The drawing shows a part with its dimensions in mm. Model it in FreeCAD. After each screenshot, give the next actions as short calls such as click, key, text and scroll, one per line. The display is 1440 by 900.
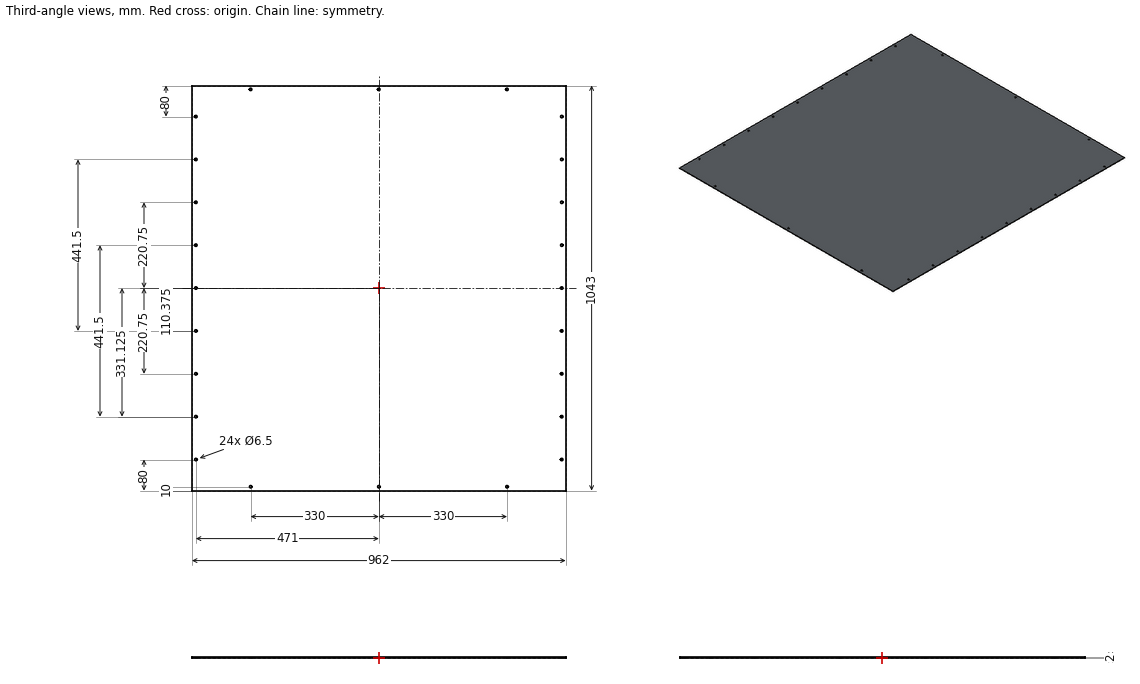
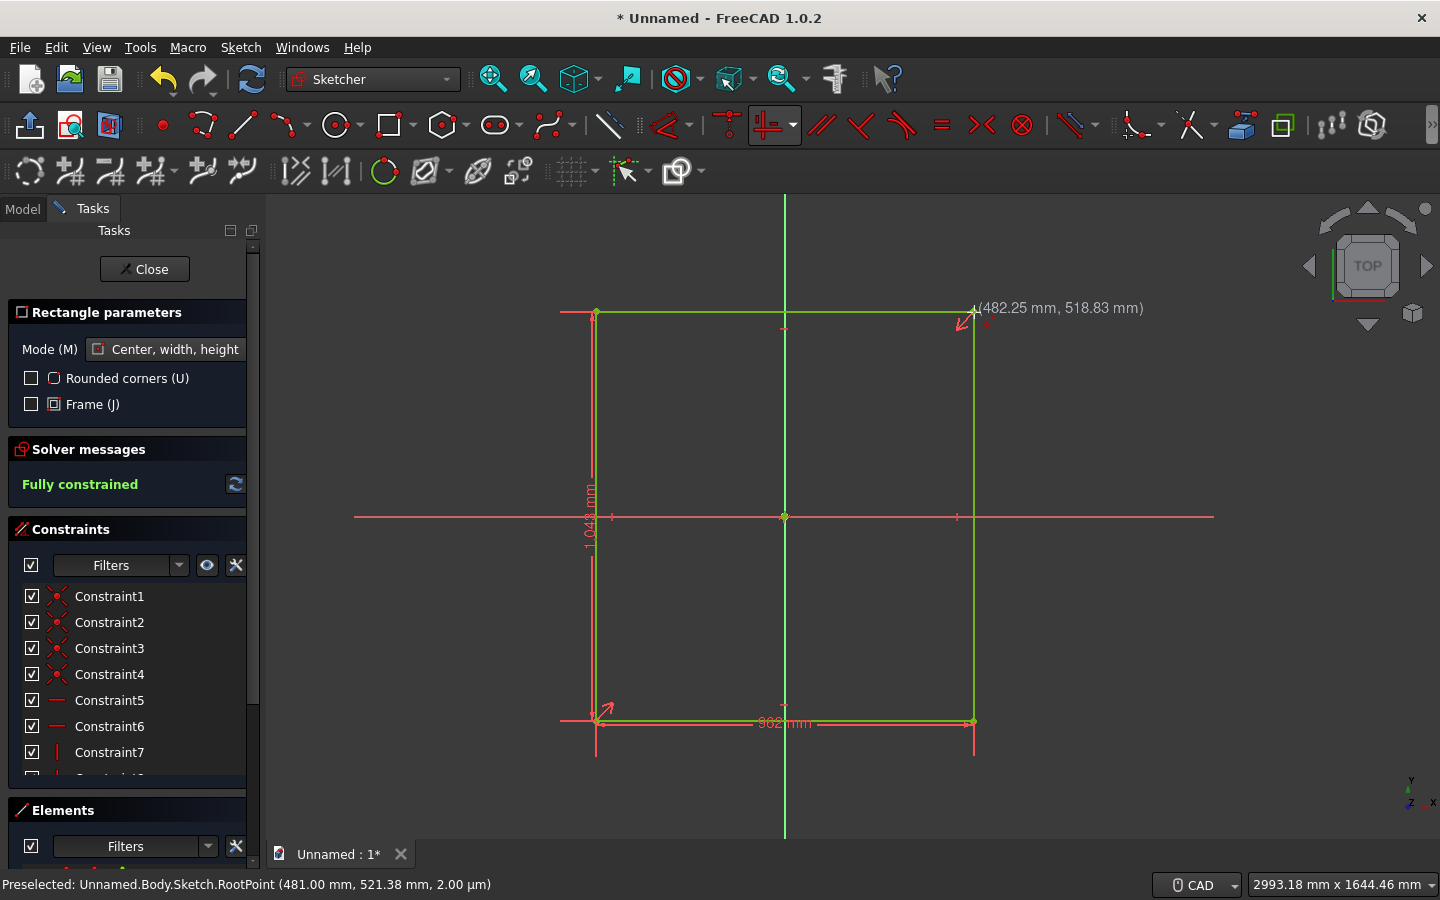
click(336, 126)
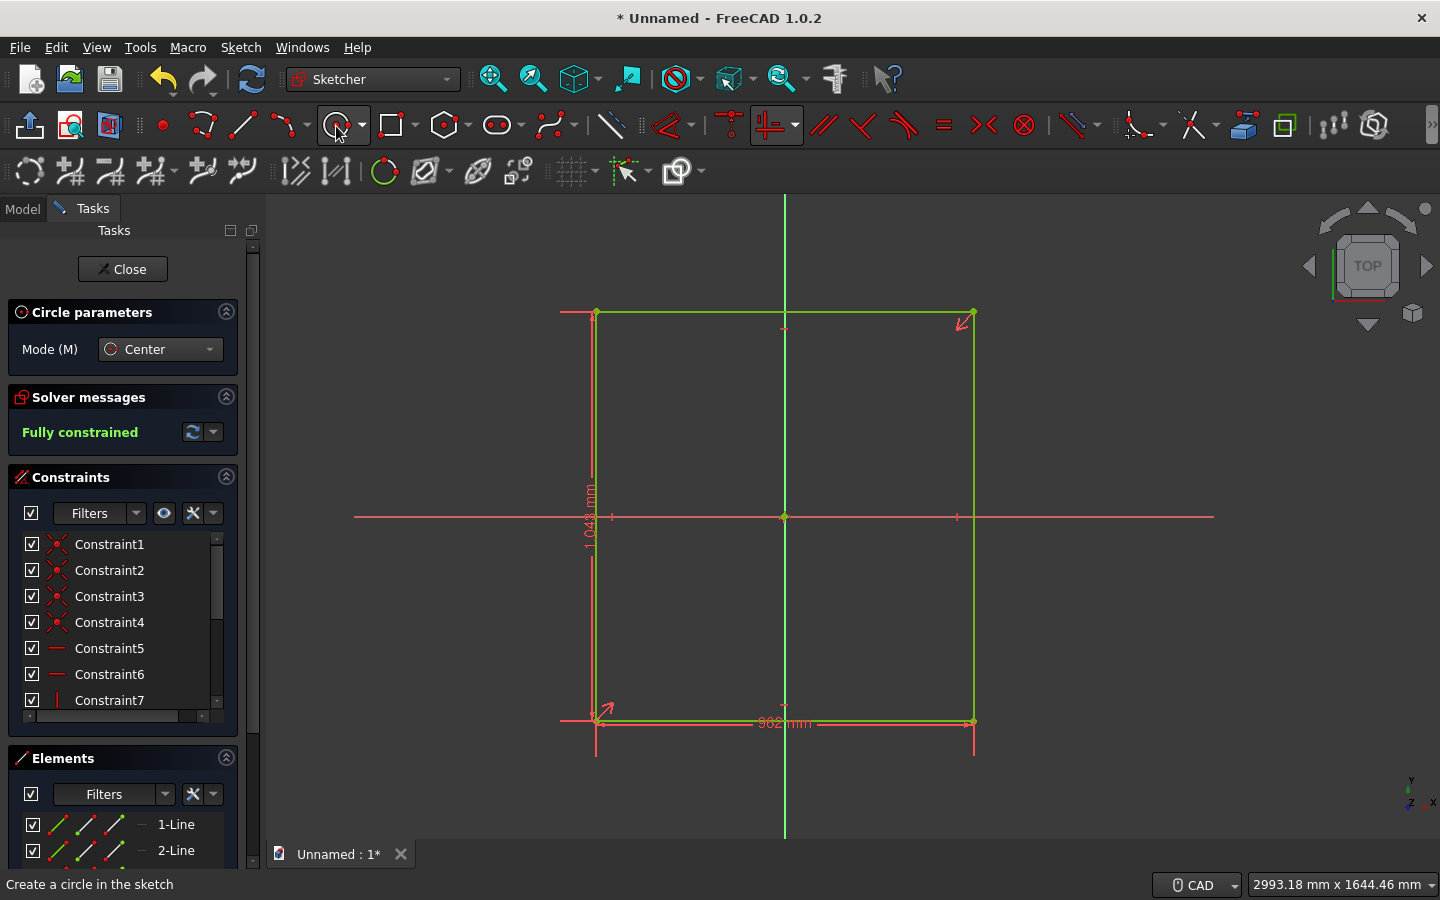
scroll(600, 690, up, 15)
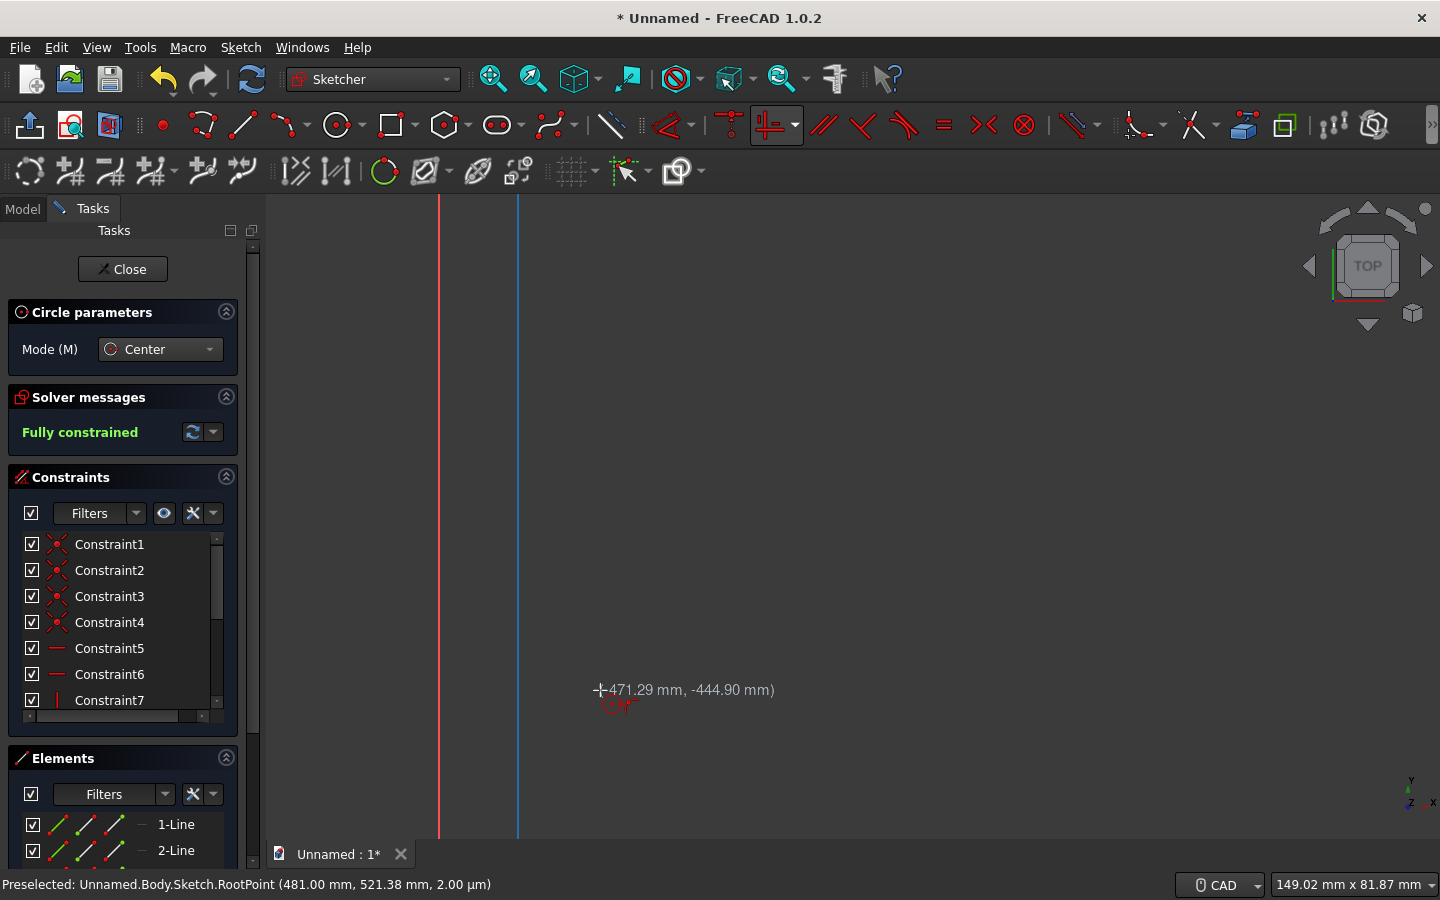
scroll(600, 691, down, 15)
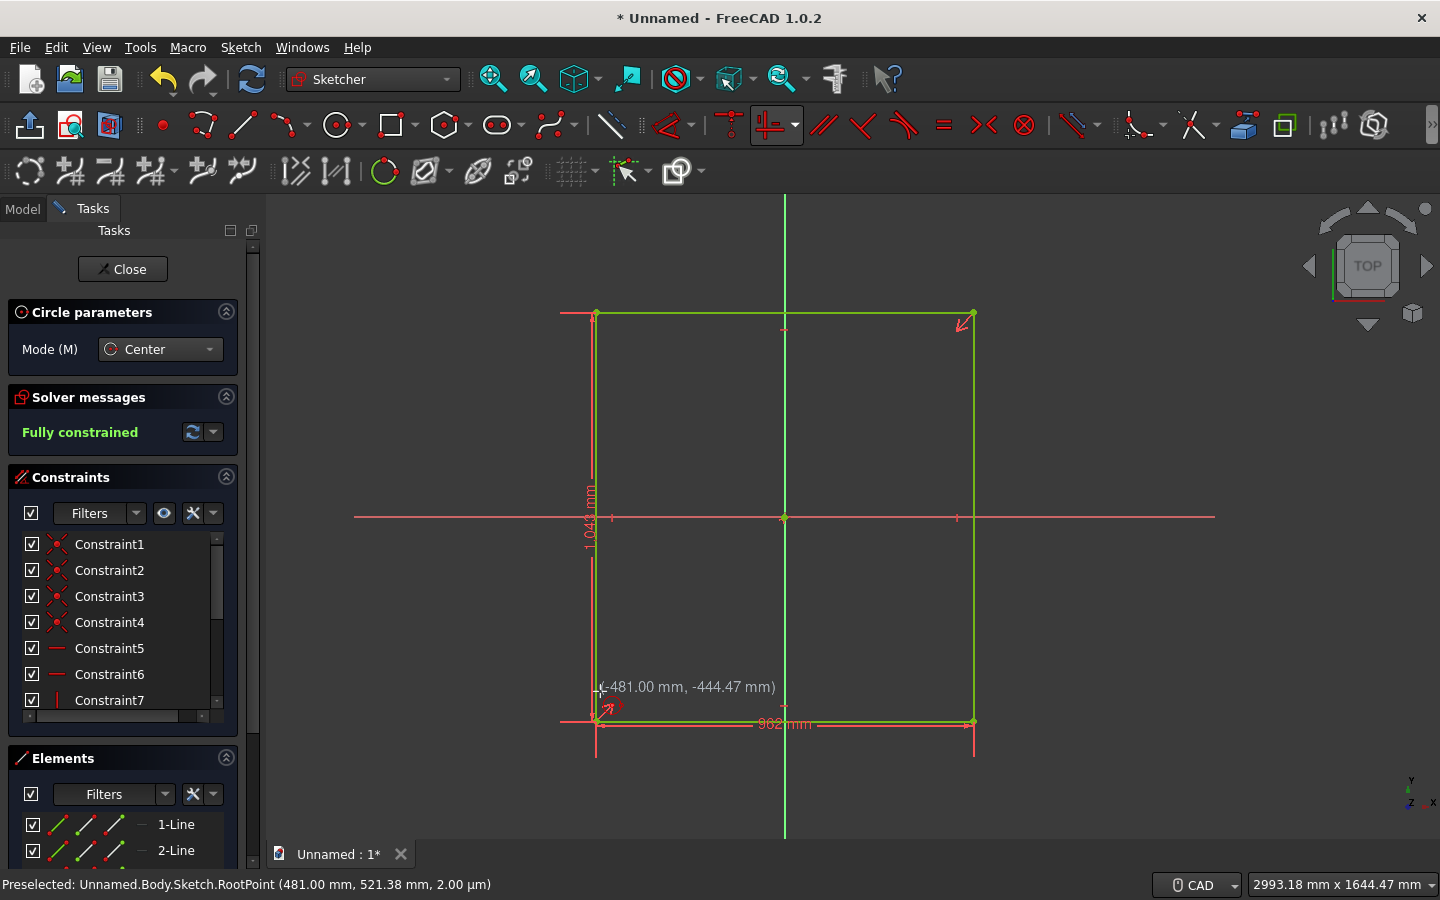
scroll(600, 691, up, 7)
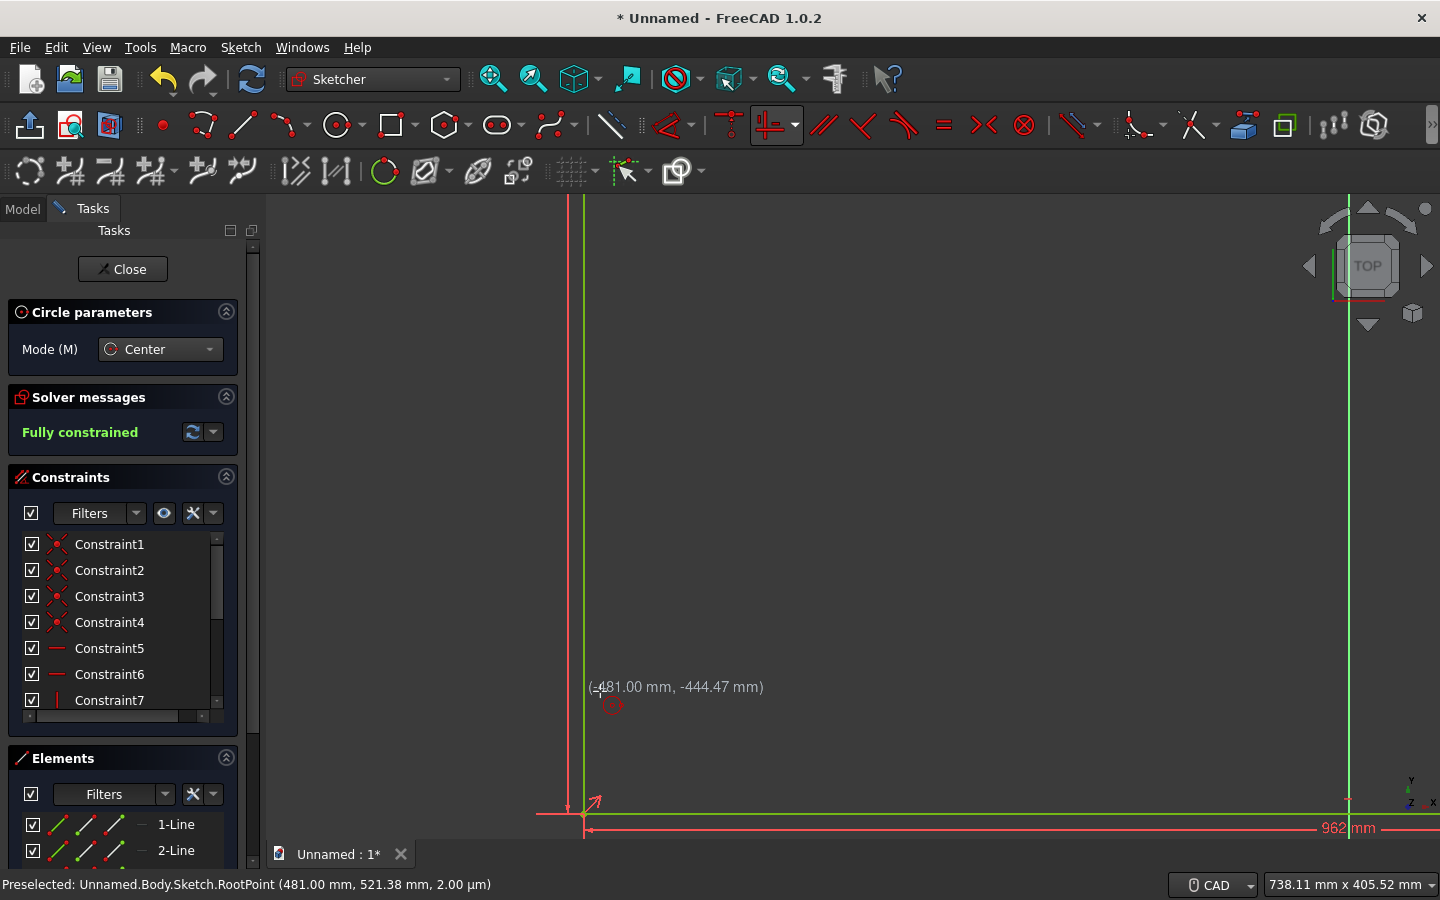
click(600, 687)
move(603, 683)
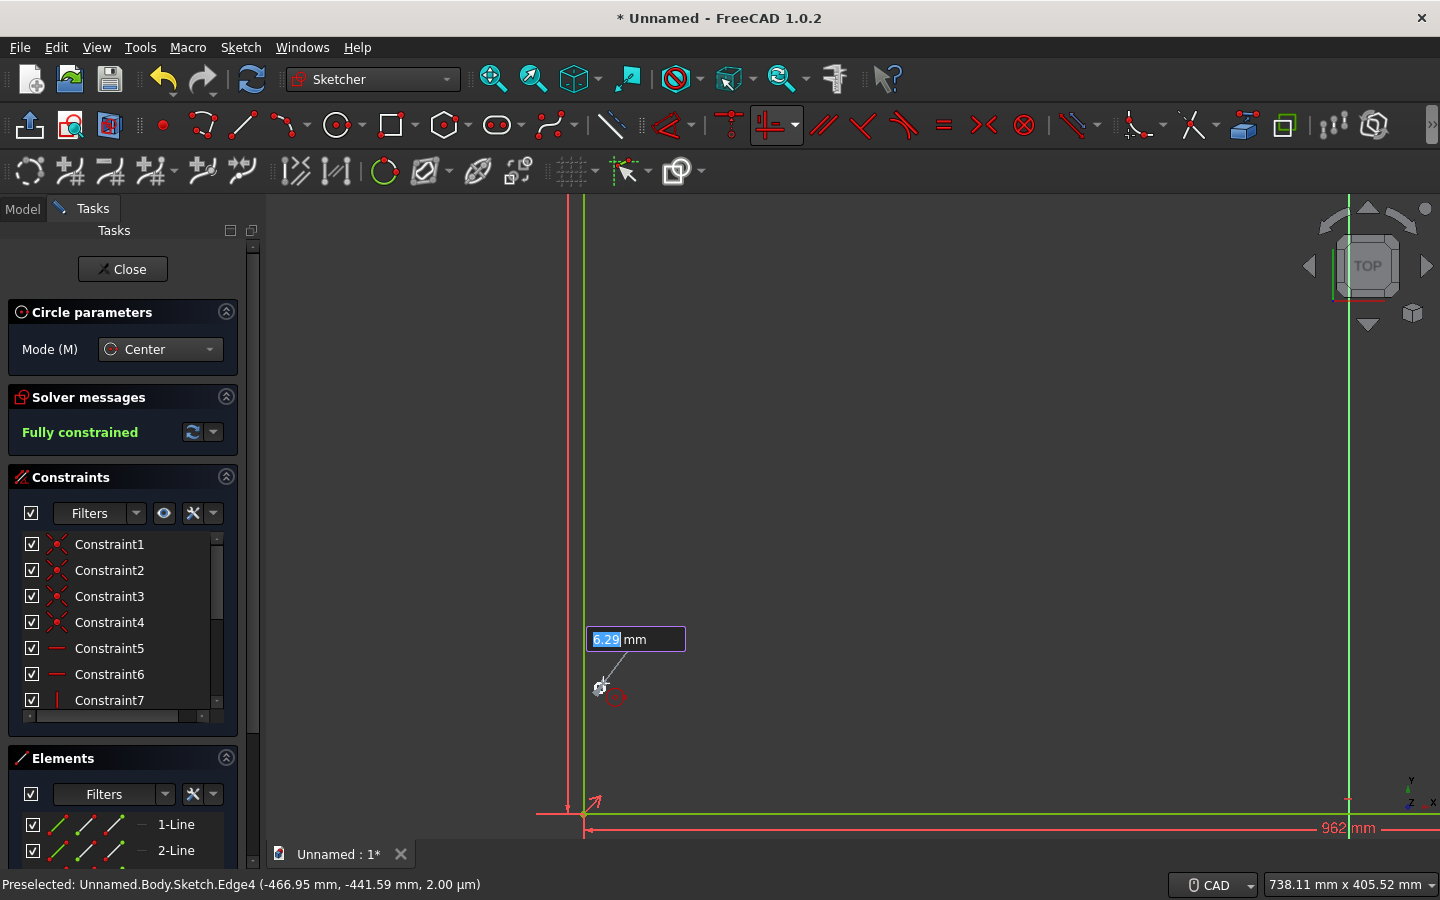
text(6.5)
key(Return)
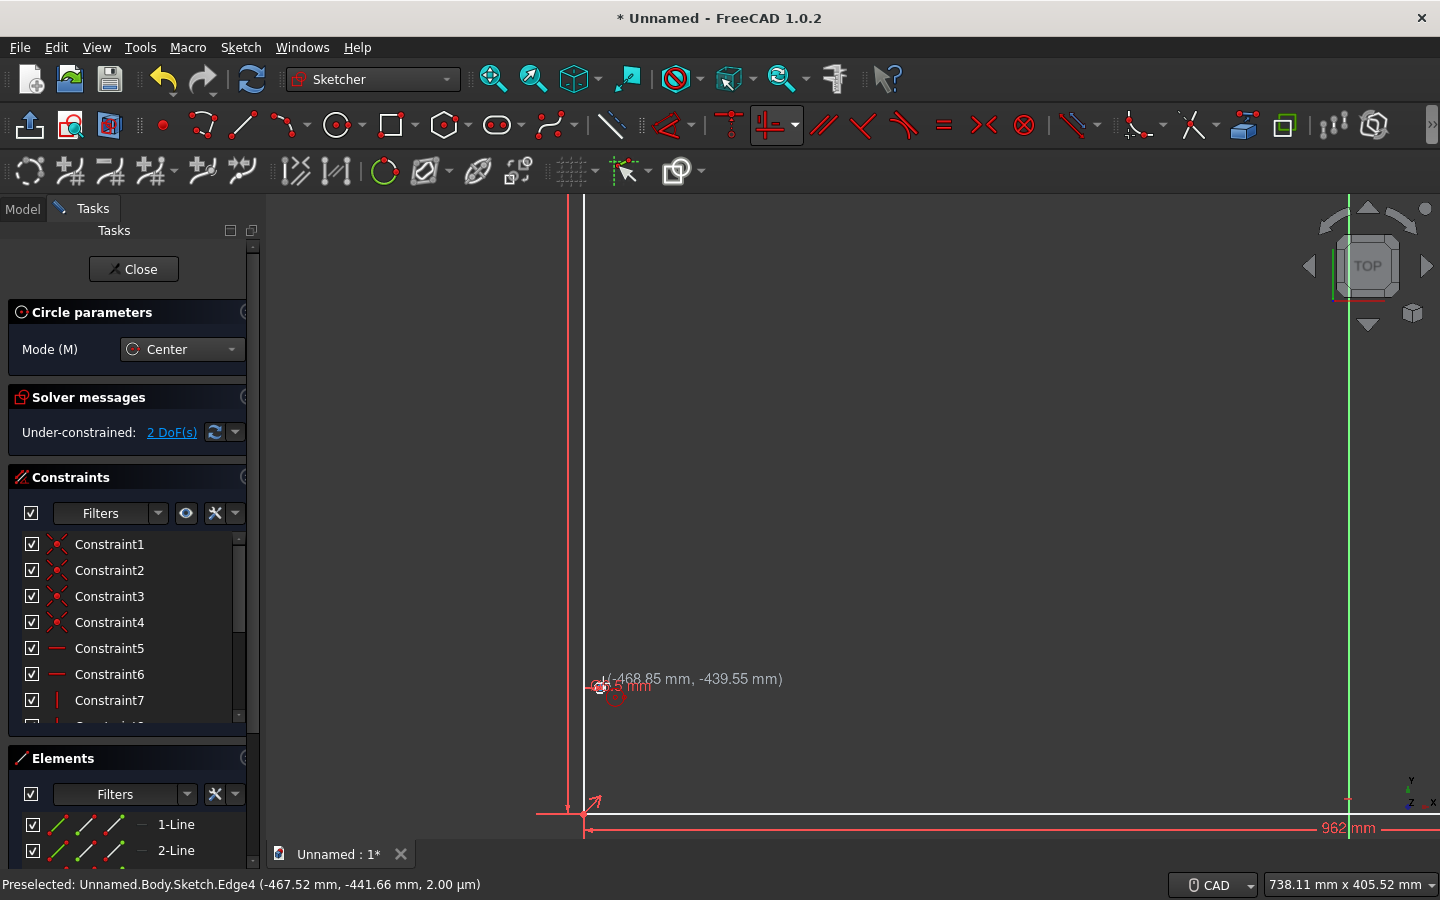
scroll(824, 798, up, 8)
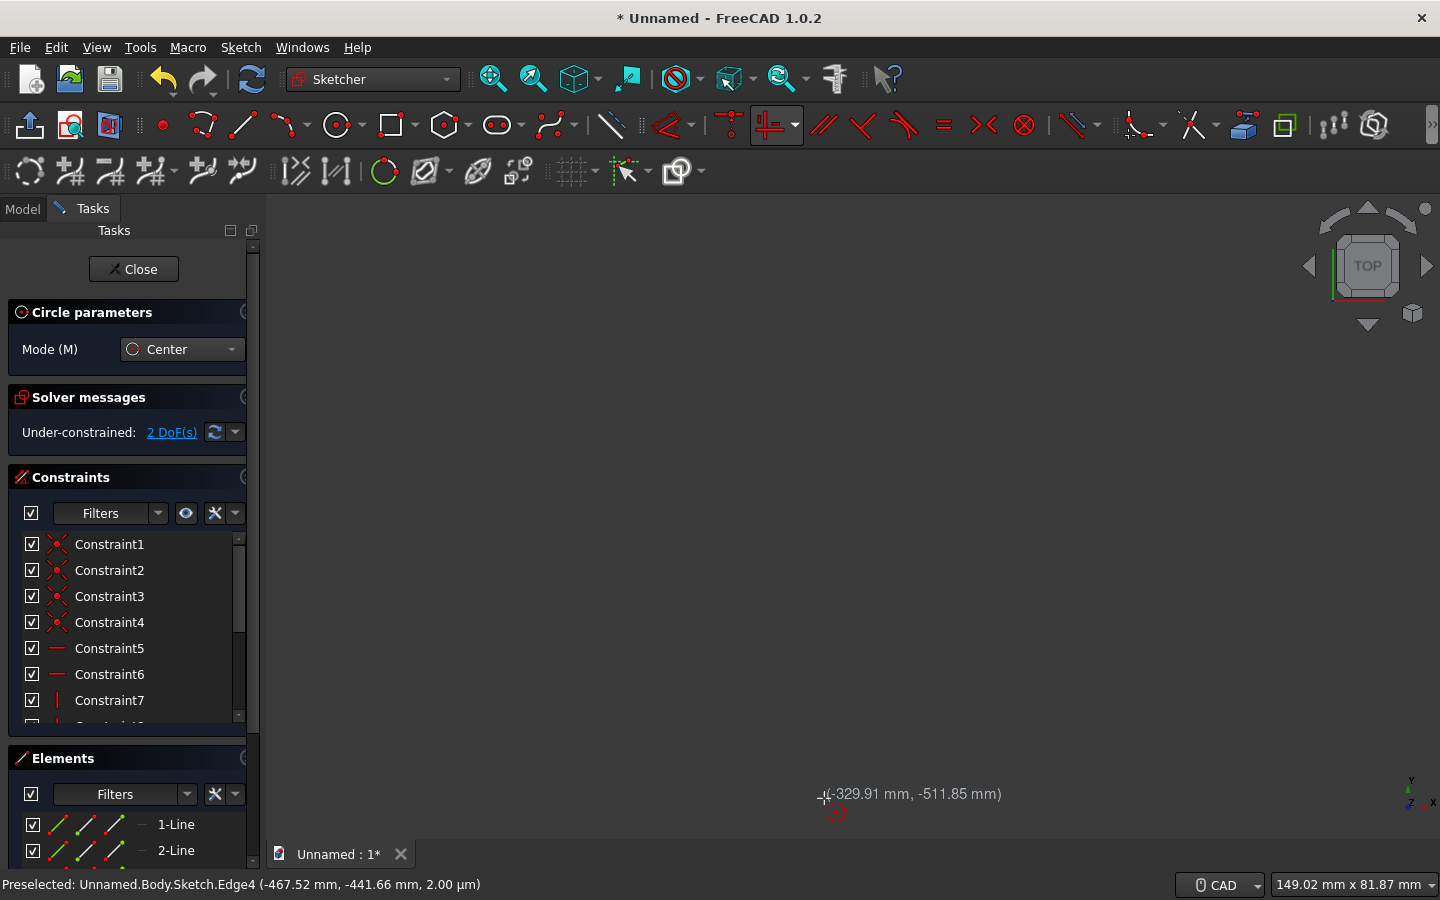
scroll(646, 713, down, 15)